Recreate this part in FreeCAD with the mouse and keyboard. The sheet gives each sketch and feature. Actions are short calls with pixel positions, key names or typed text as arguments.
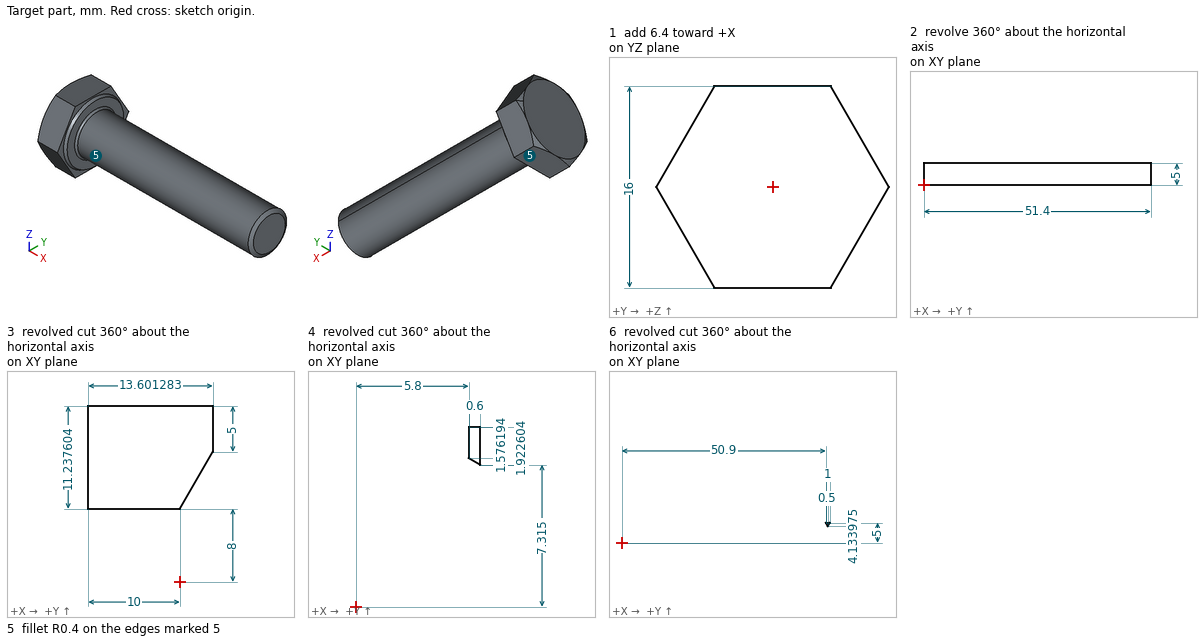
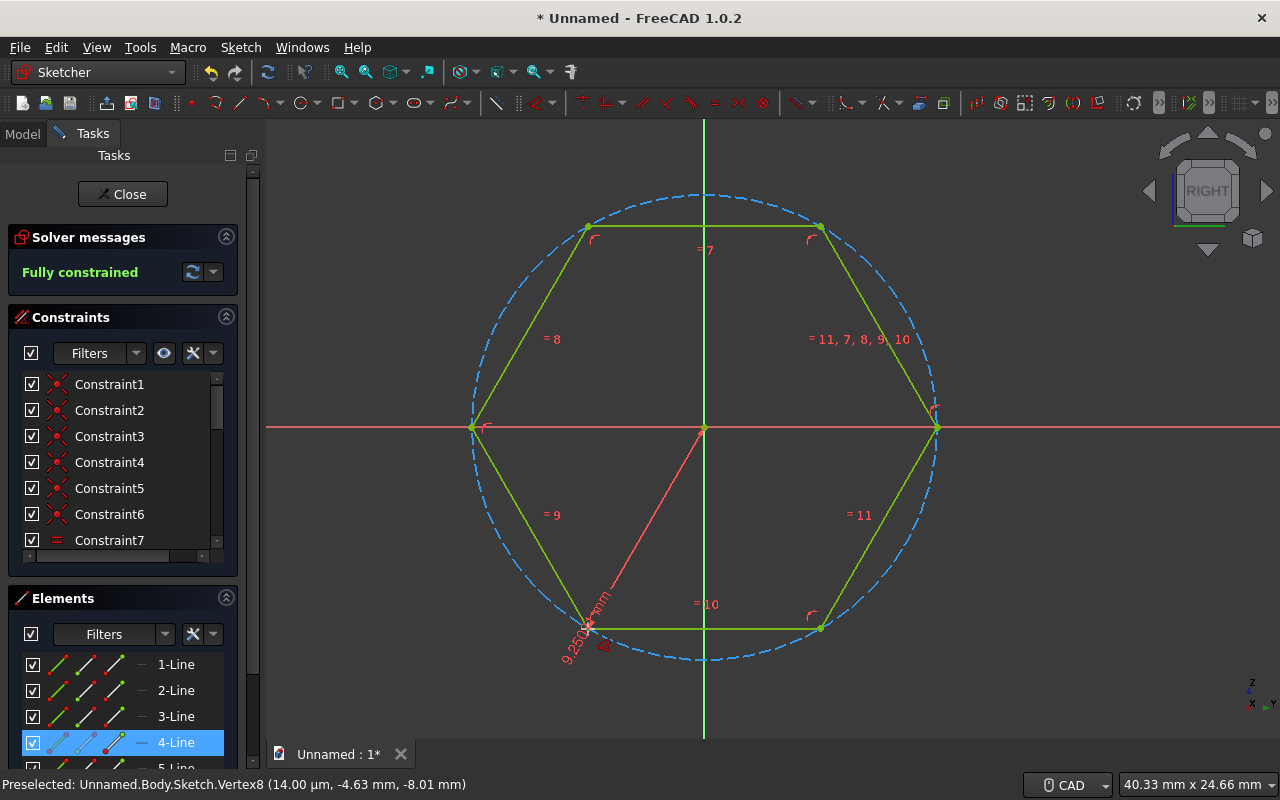
click(821, 226)
click(855, 335)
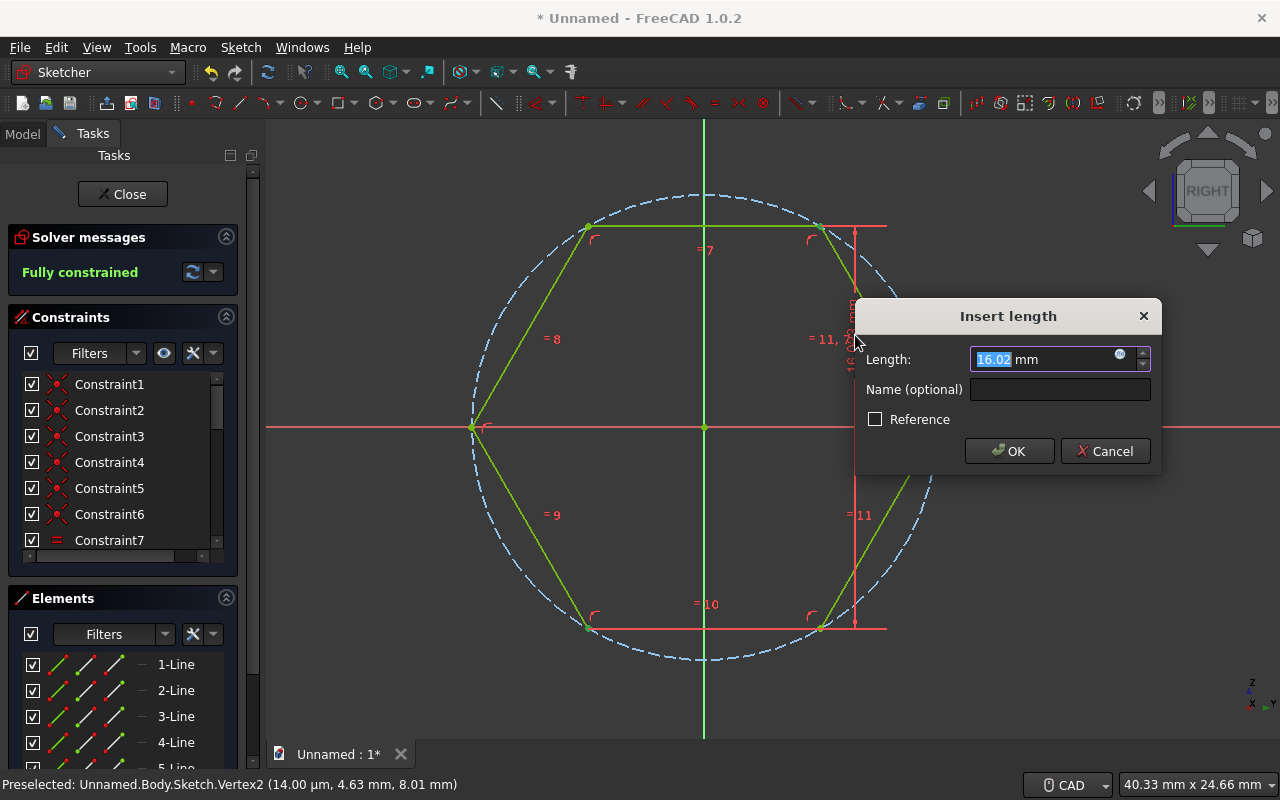
text(16)
key(Return)
key(Escape)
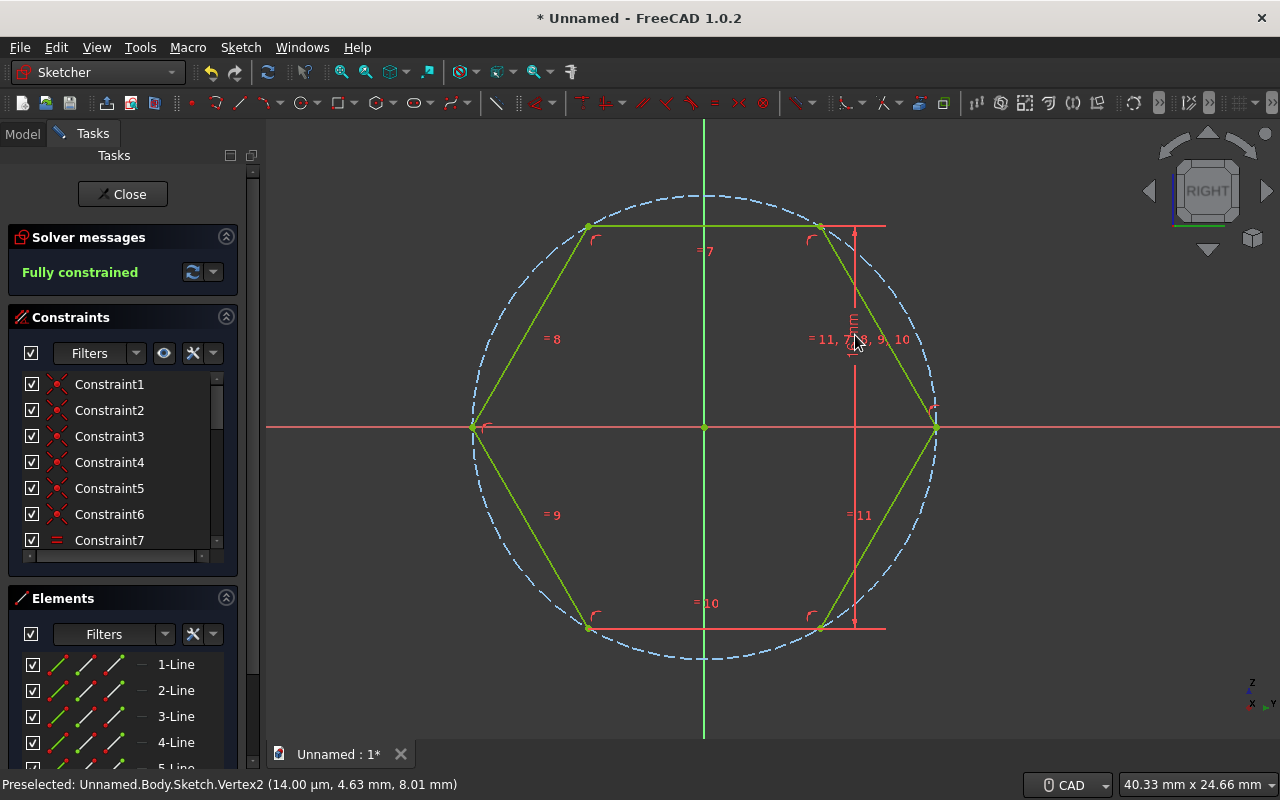
click(123, 194)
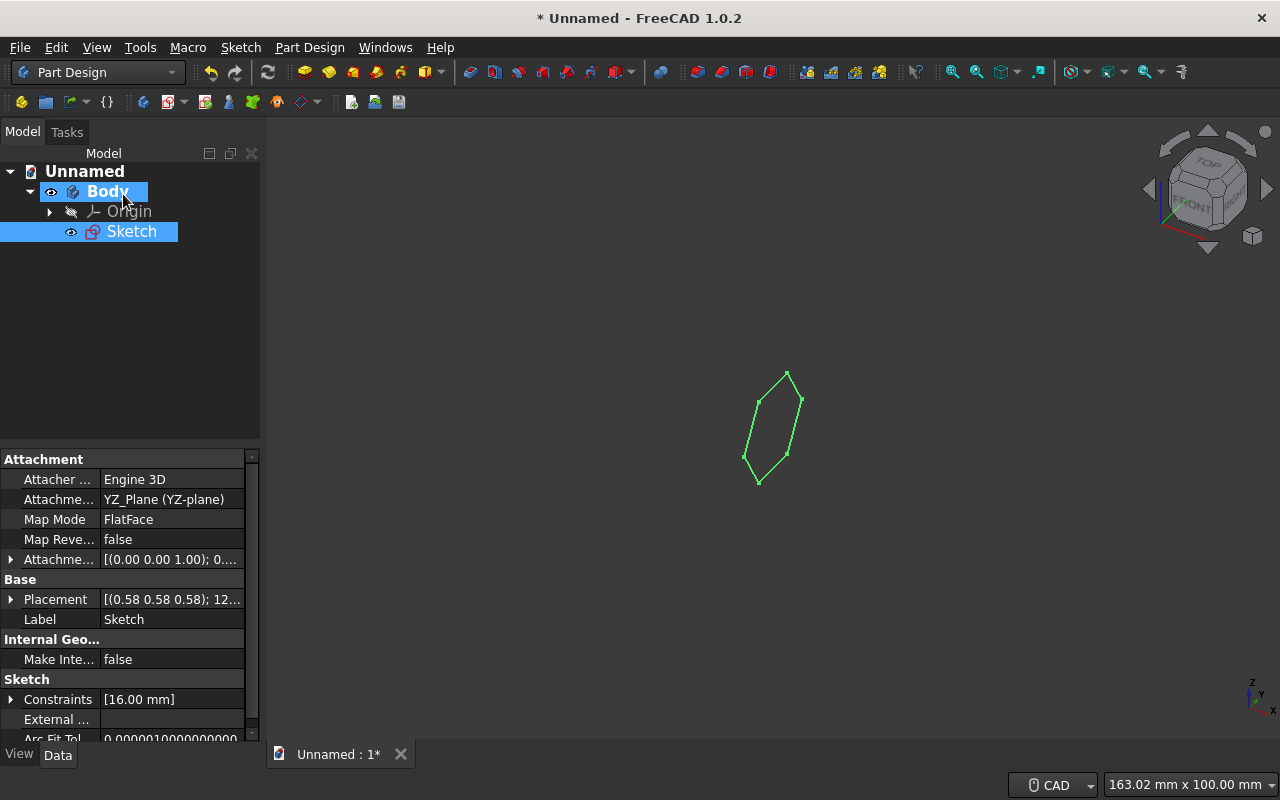
click(306, 72)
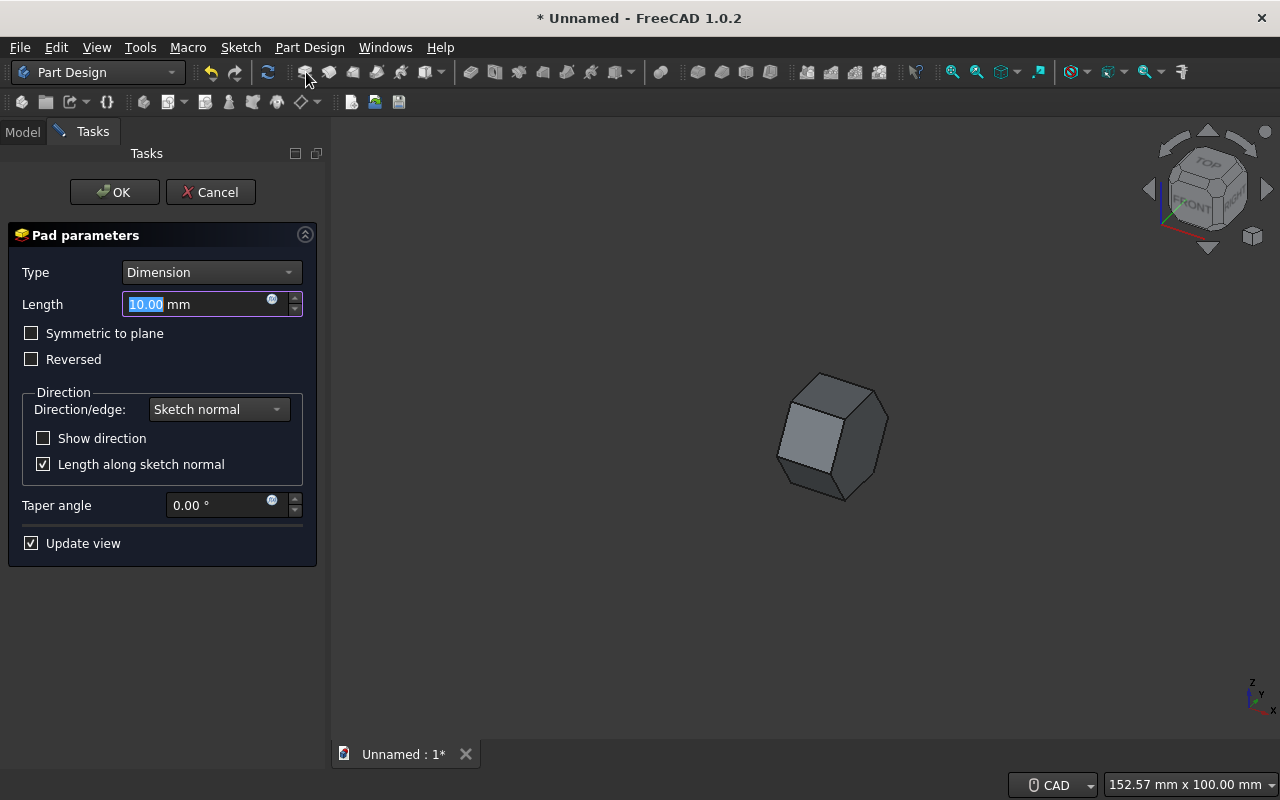
text(6.4)
key(Tab)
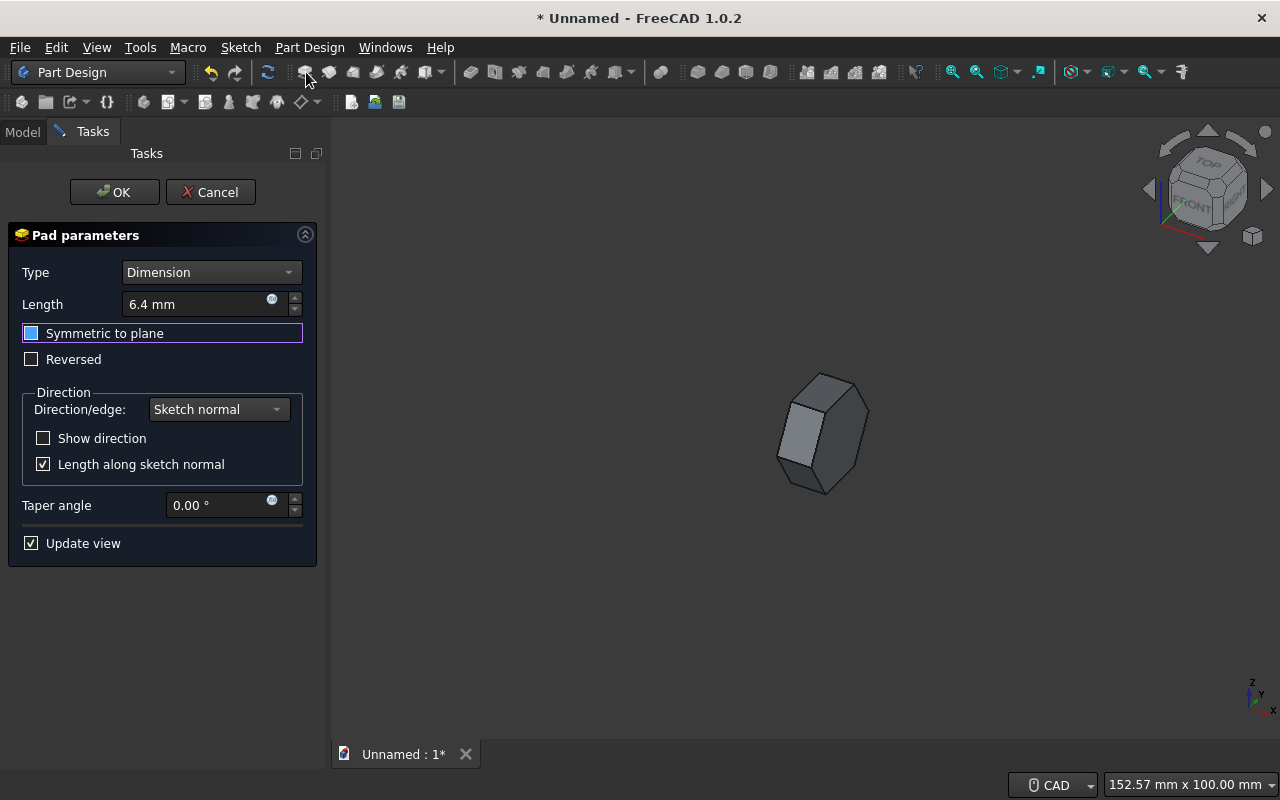
click(115, 192)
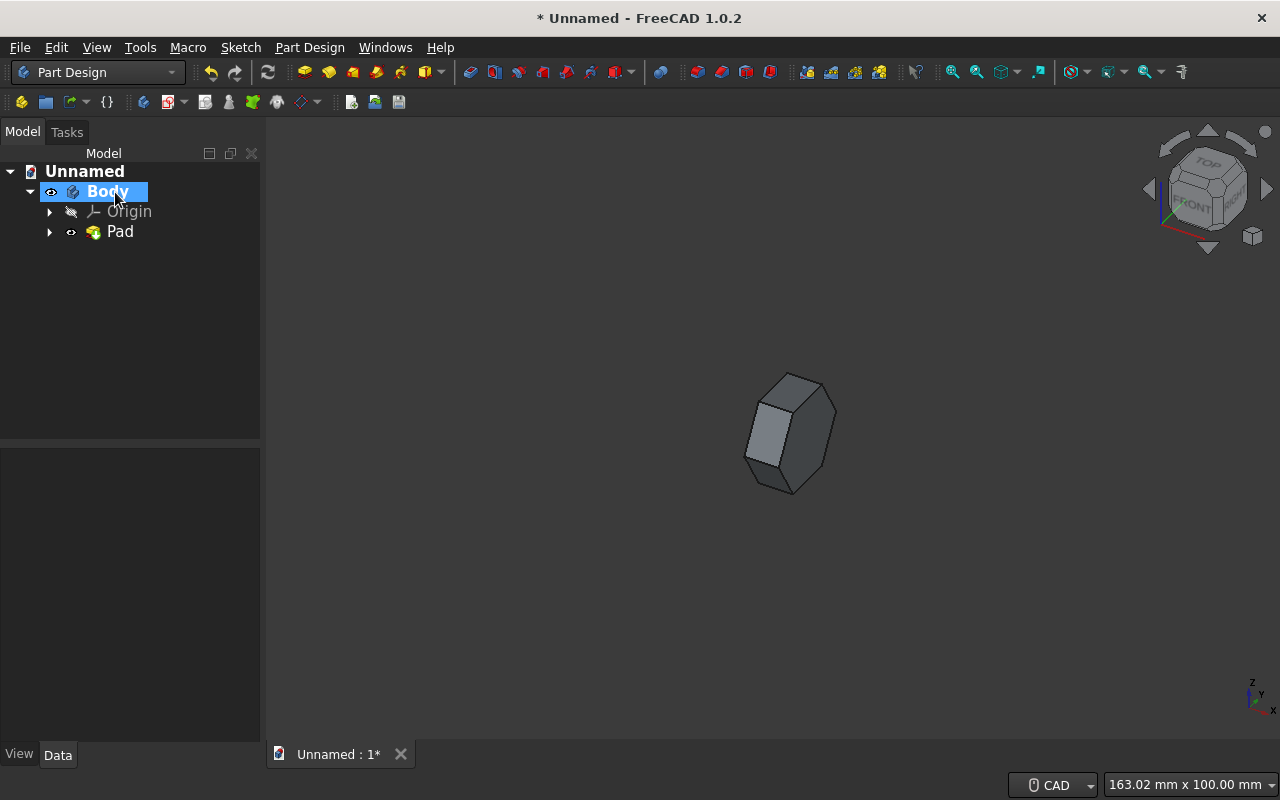
click(954, 72)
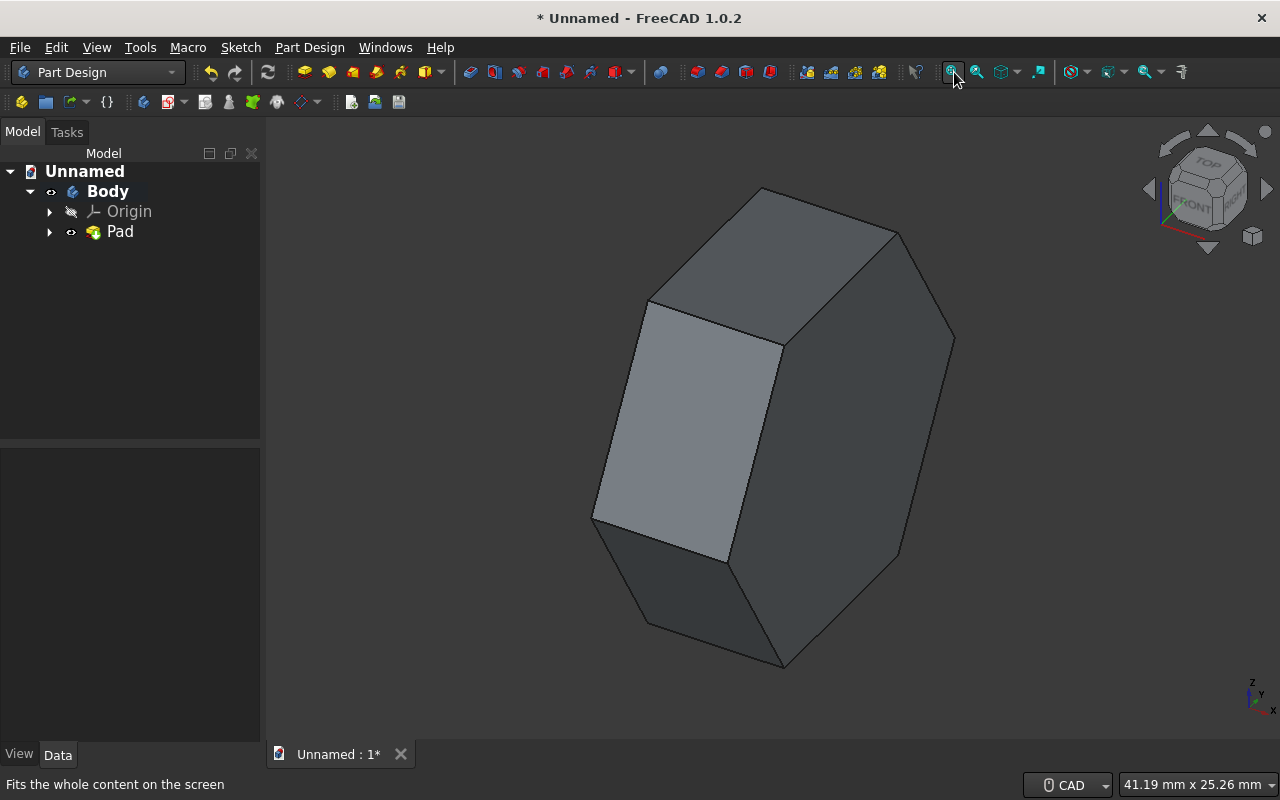
click(168, 102)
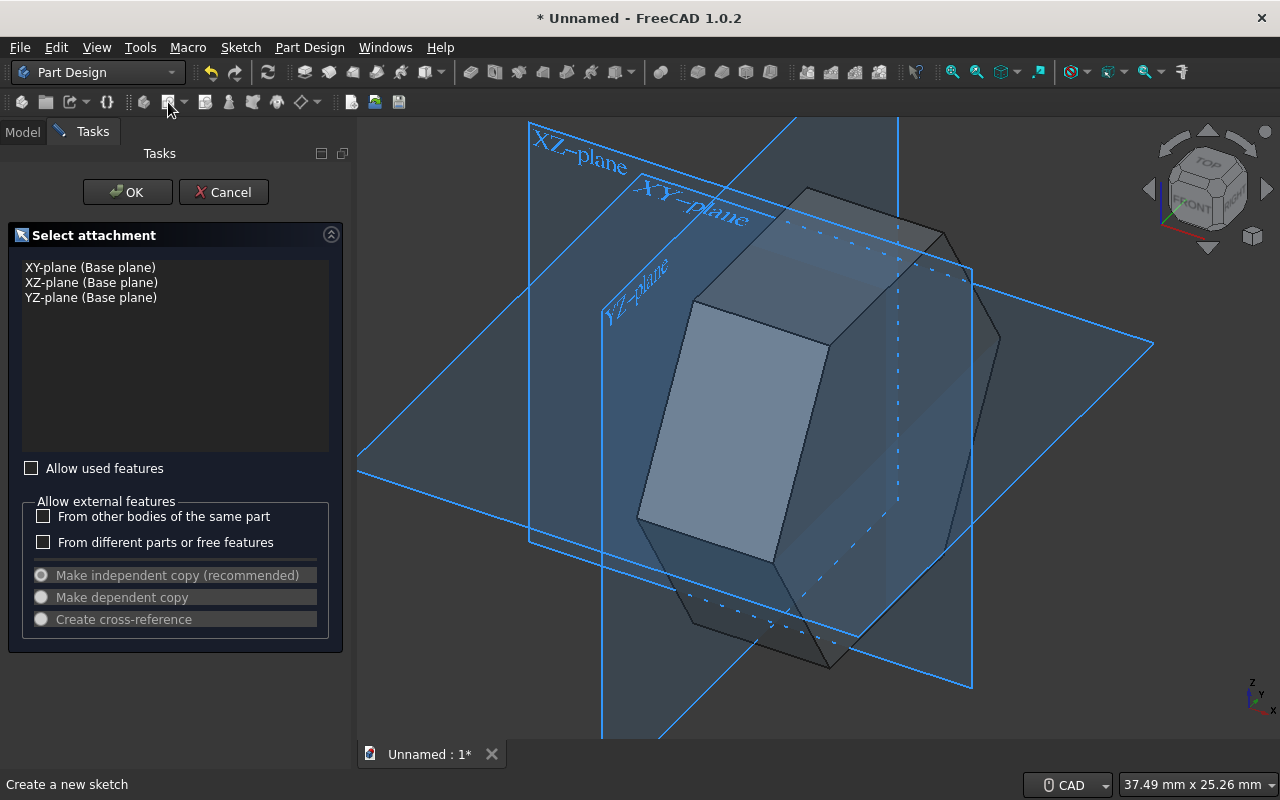
click(82, 268)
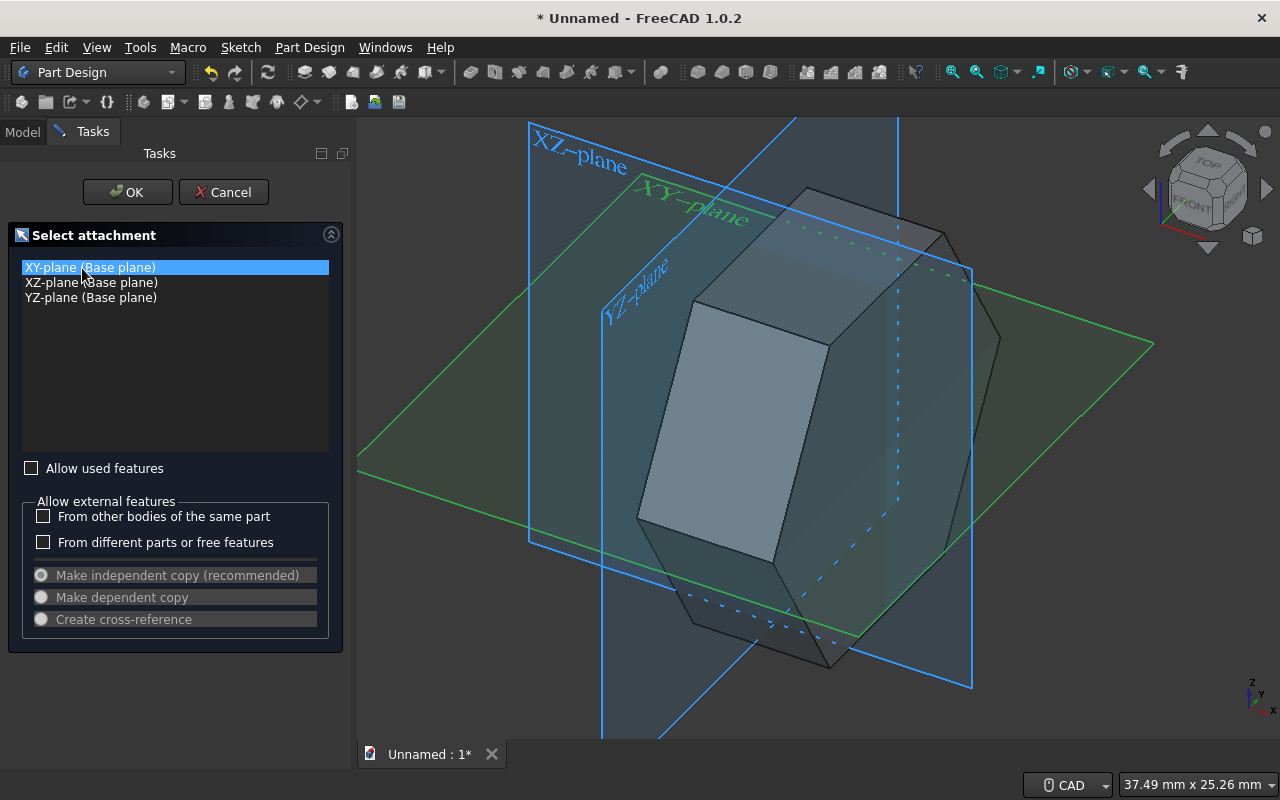
click(128, 192)